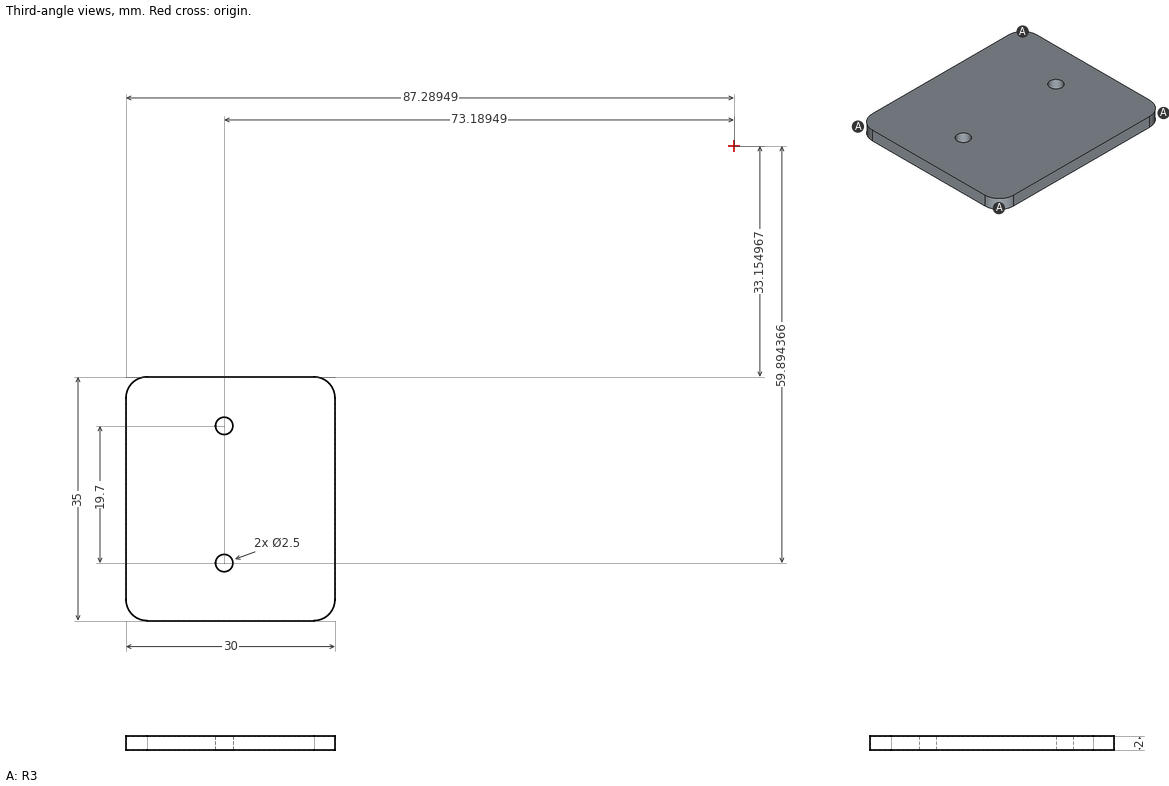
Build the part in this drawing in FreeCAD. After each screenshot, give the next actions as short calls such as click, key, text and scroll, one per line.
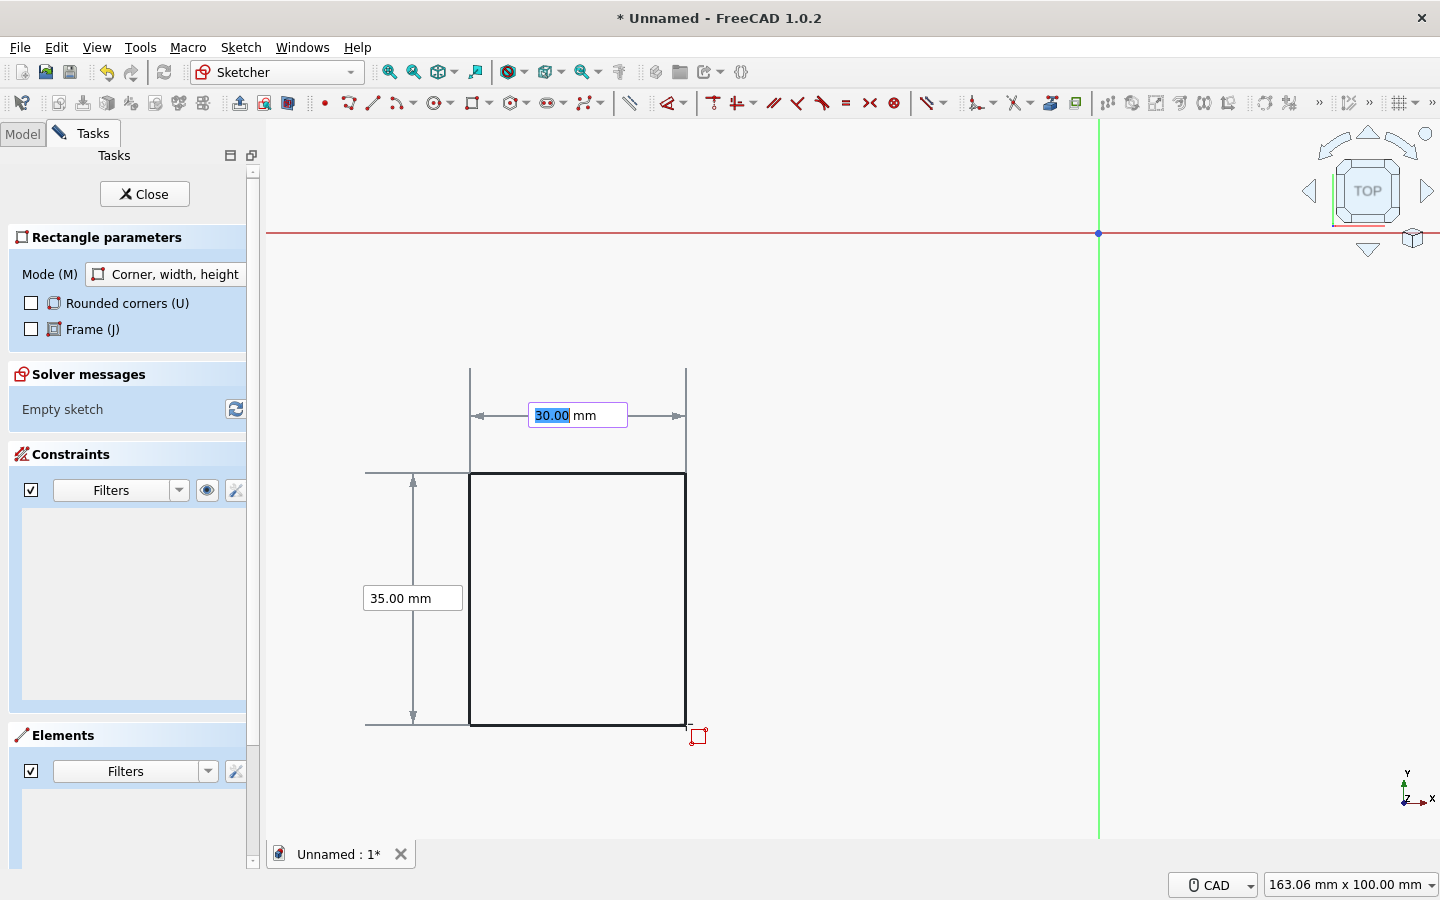
text(30)
key(Tab)
text(35)
key(Return)
key(Escape)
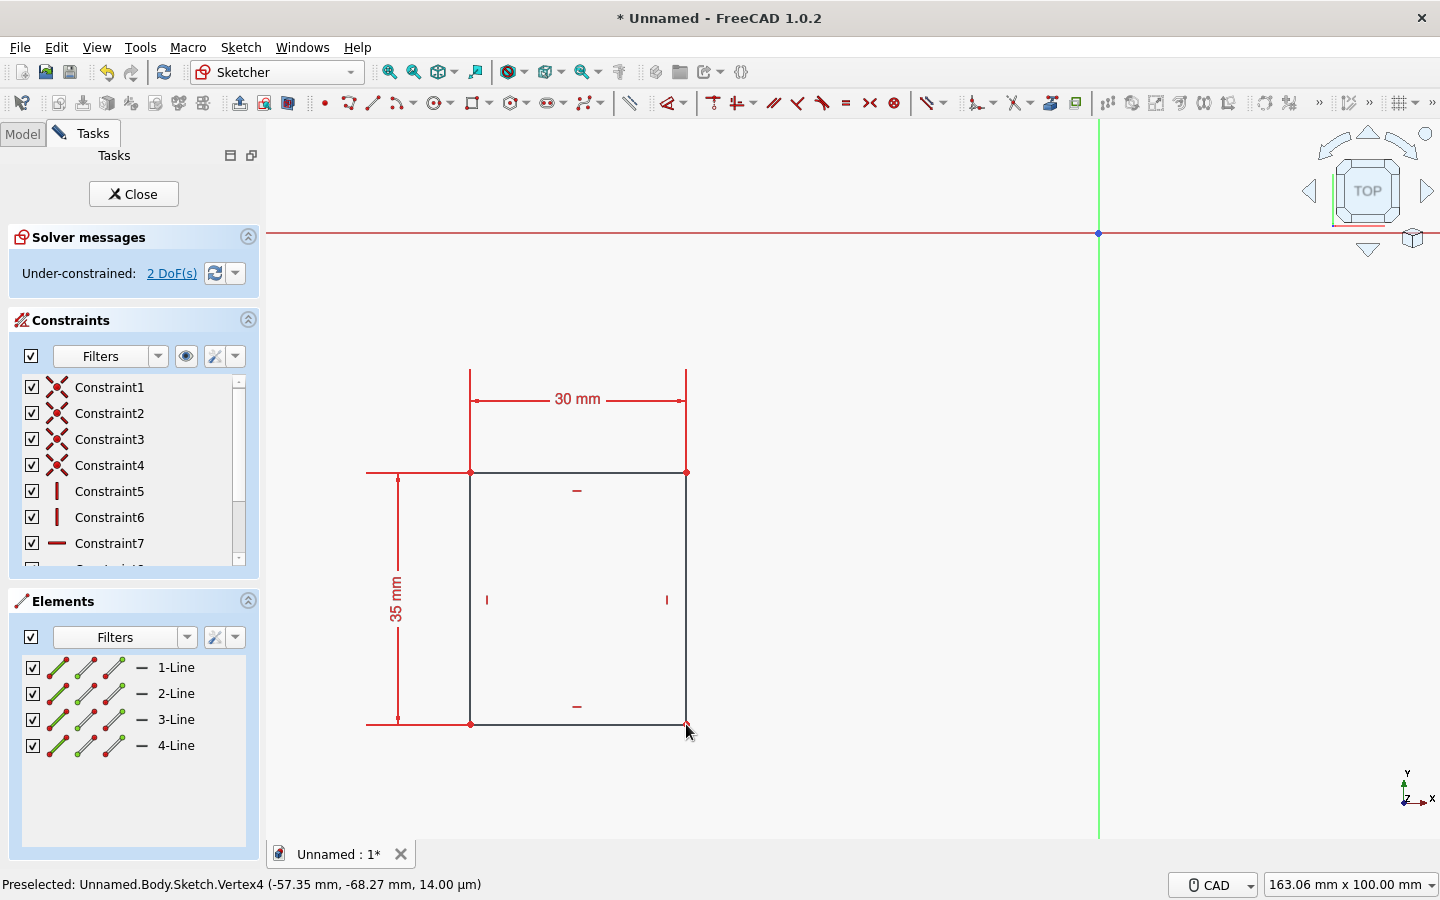
click(470, 473)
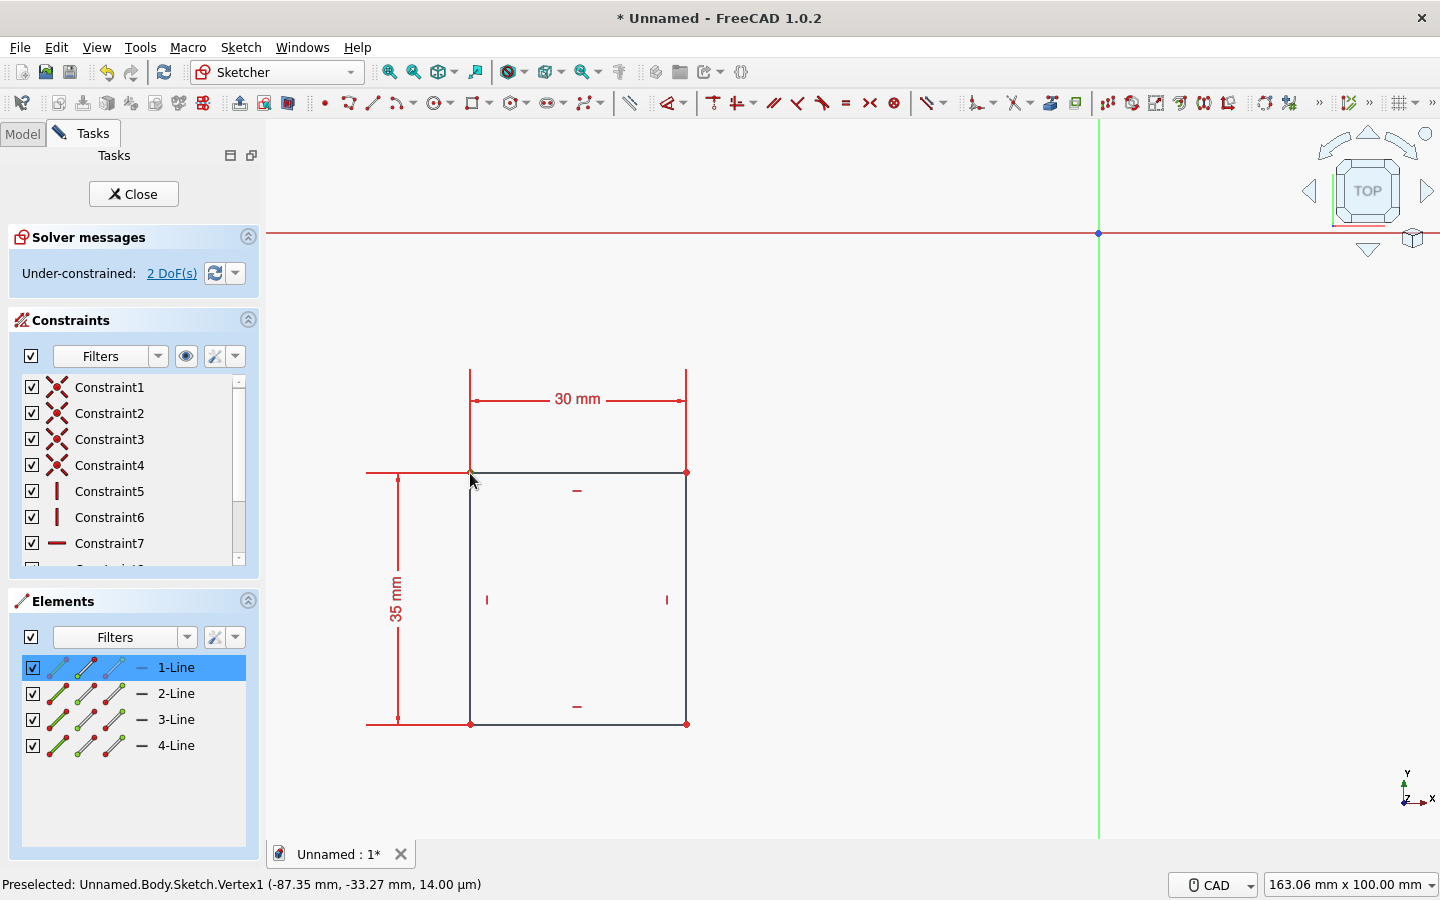
key(l)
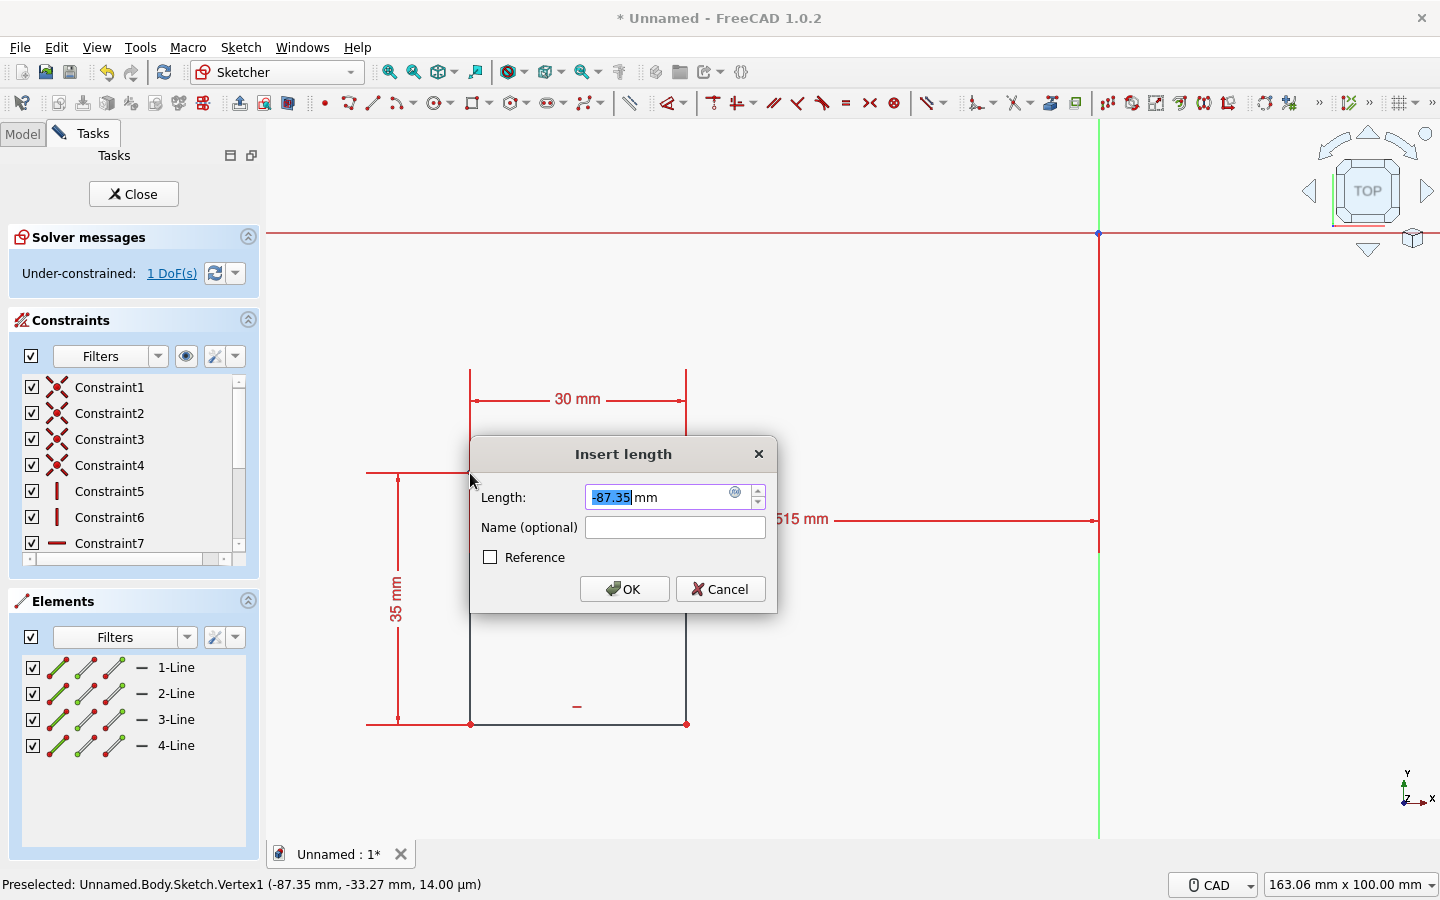
text(-87.28949)
key(Return)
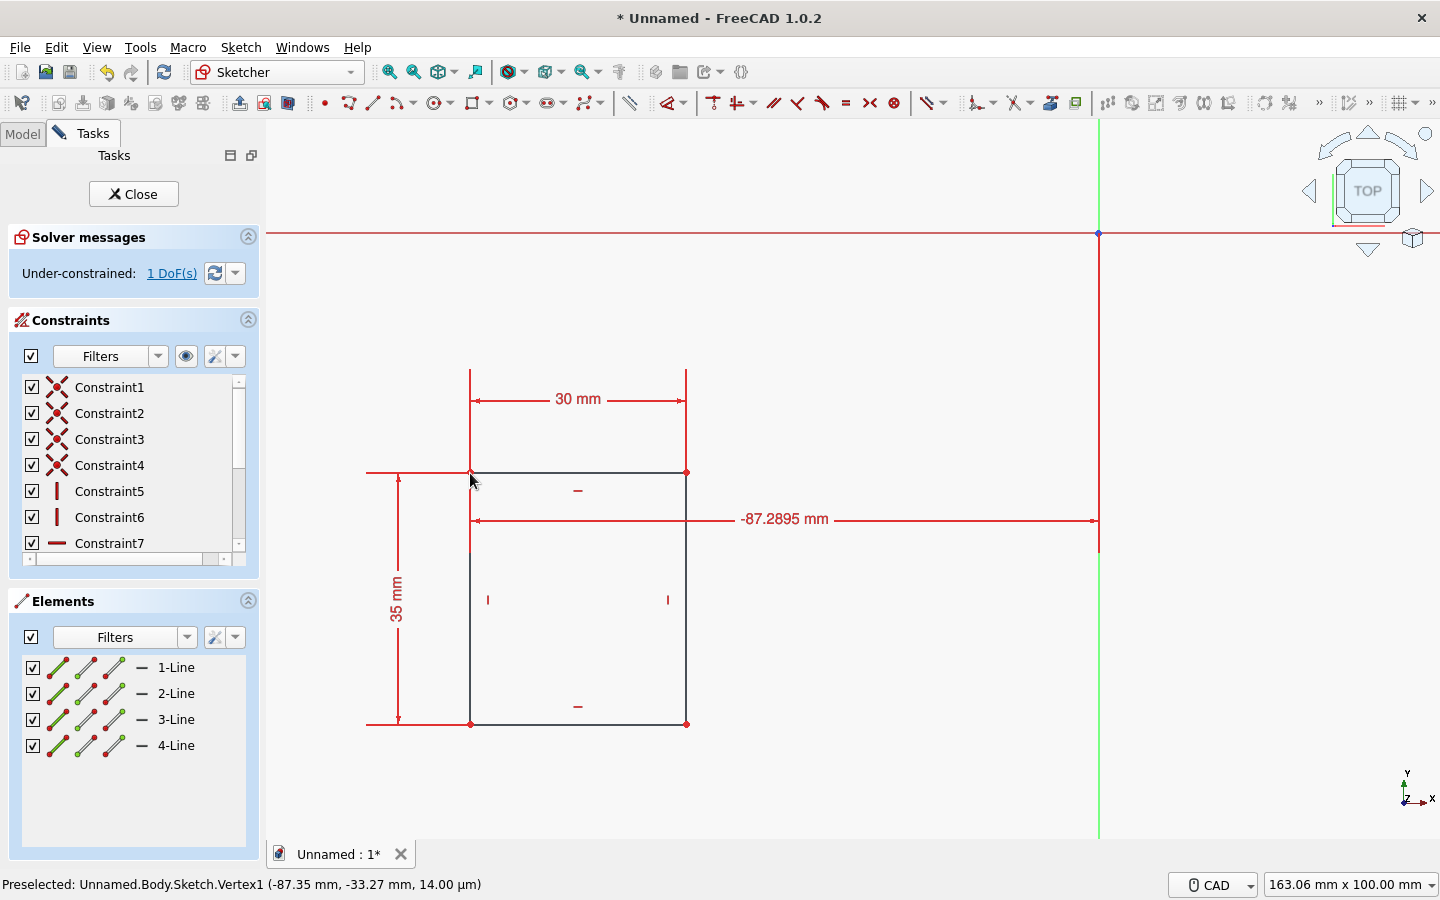
click(470, 473)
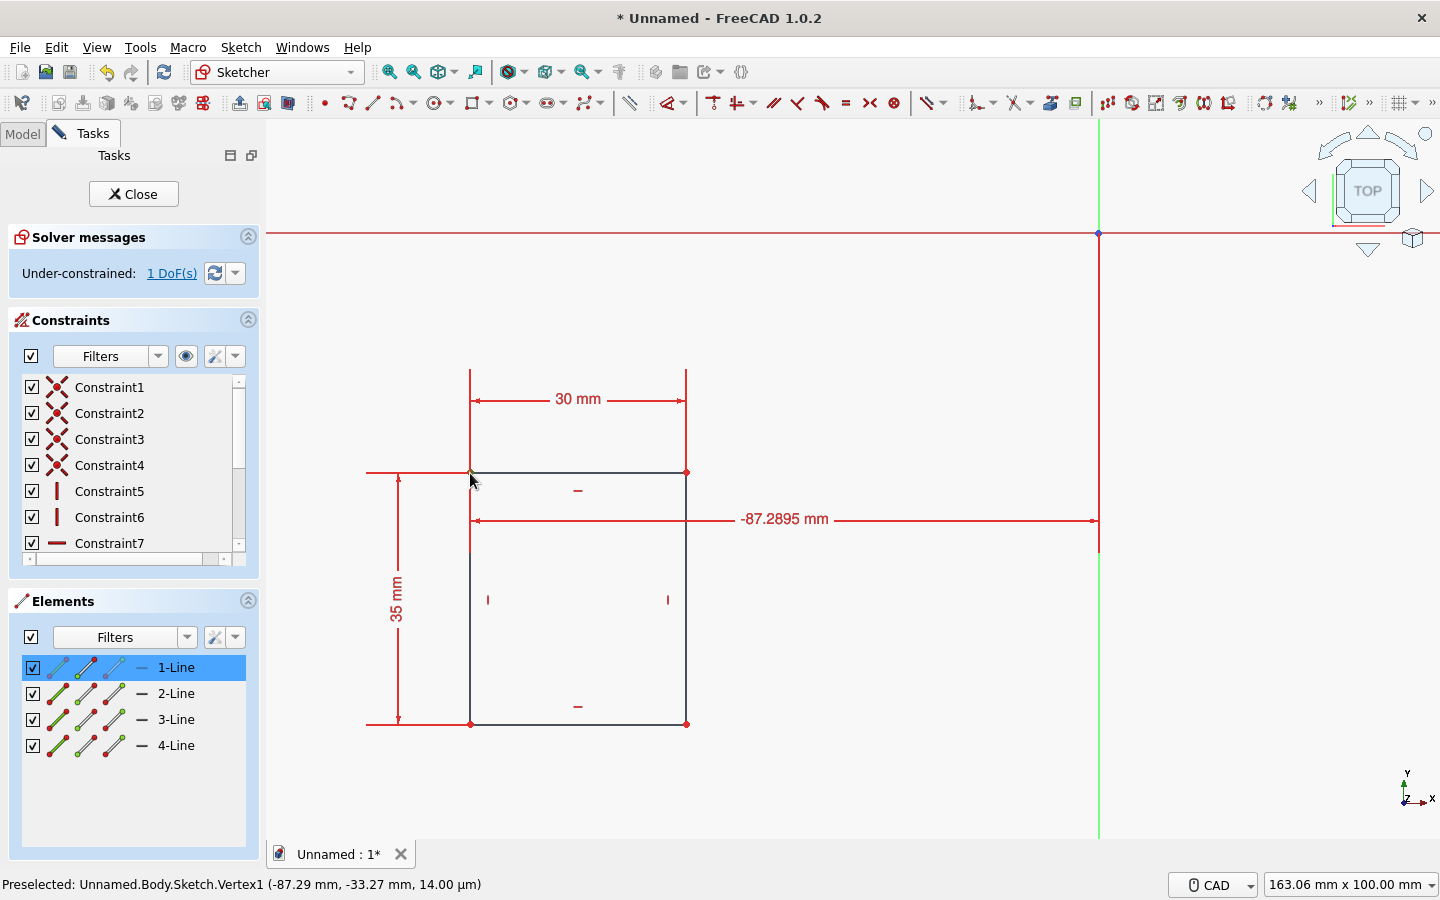
key(i)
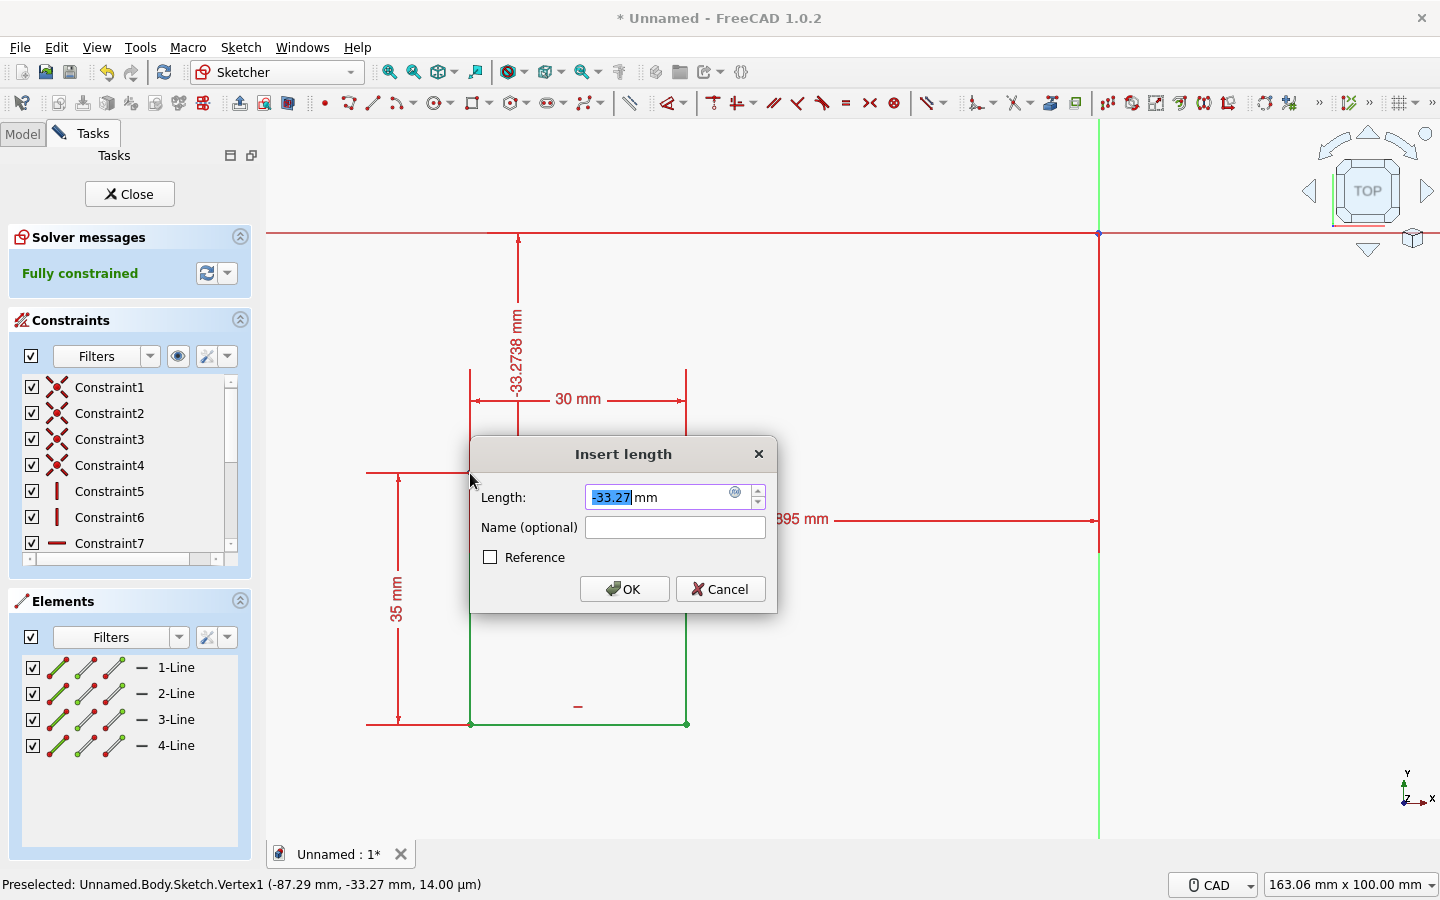
text(-33.154967)
key(Return)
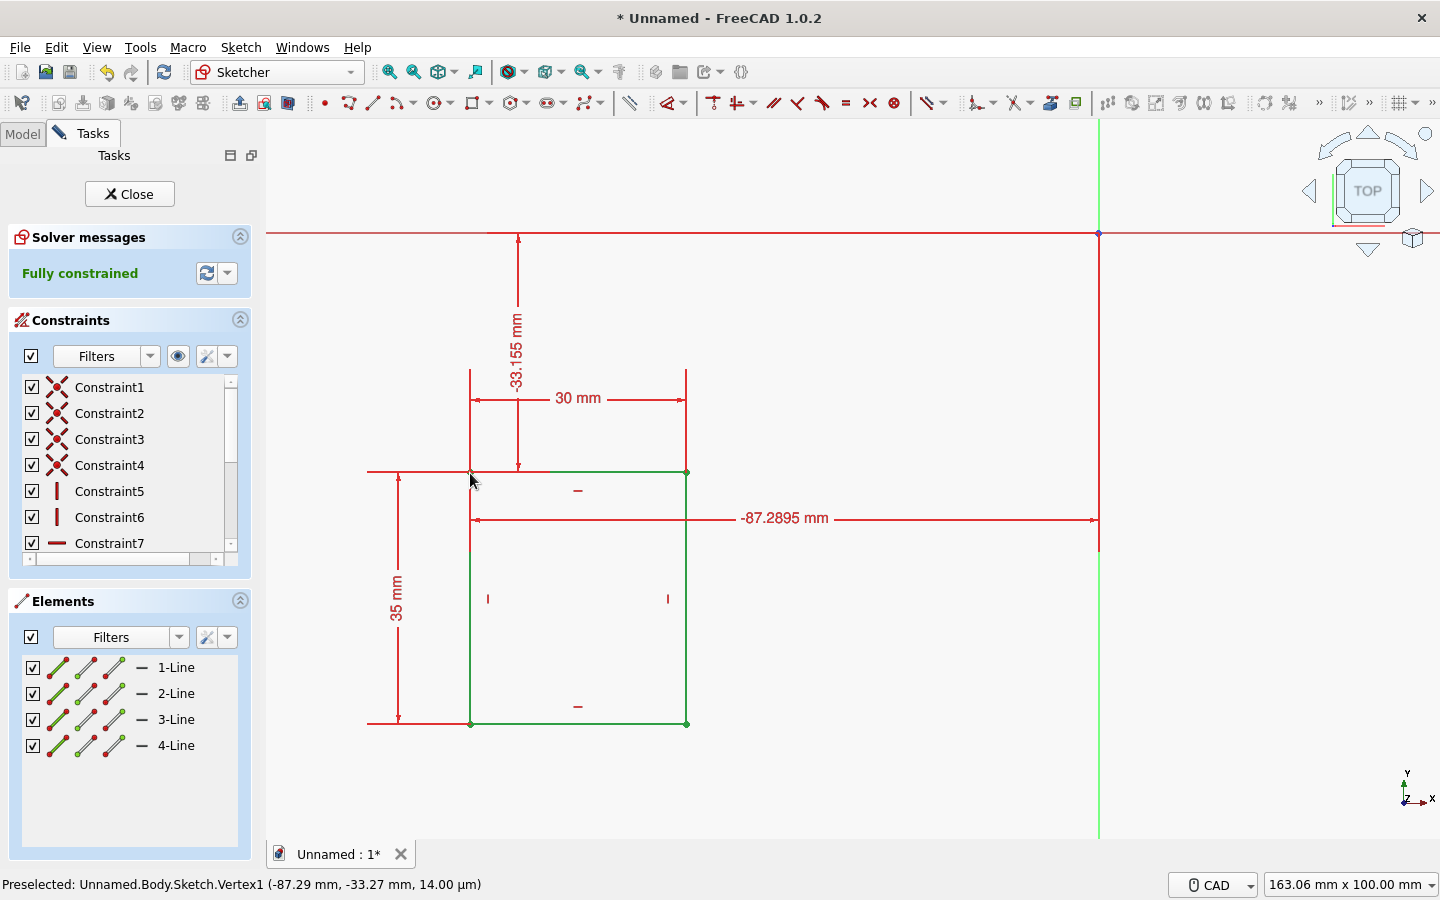
click(130, 194)